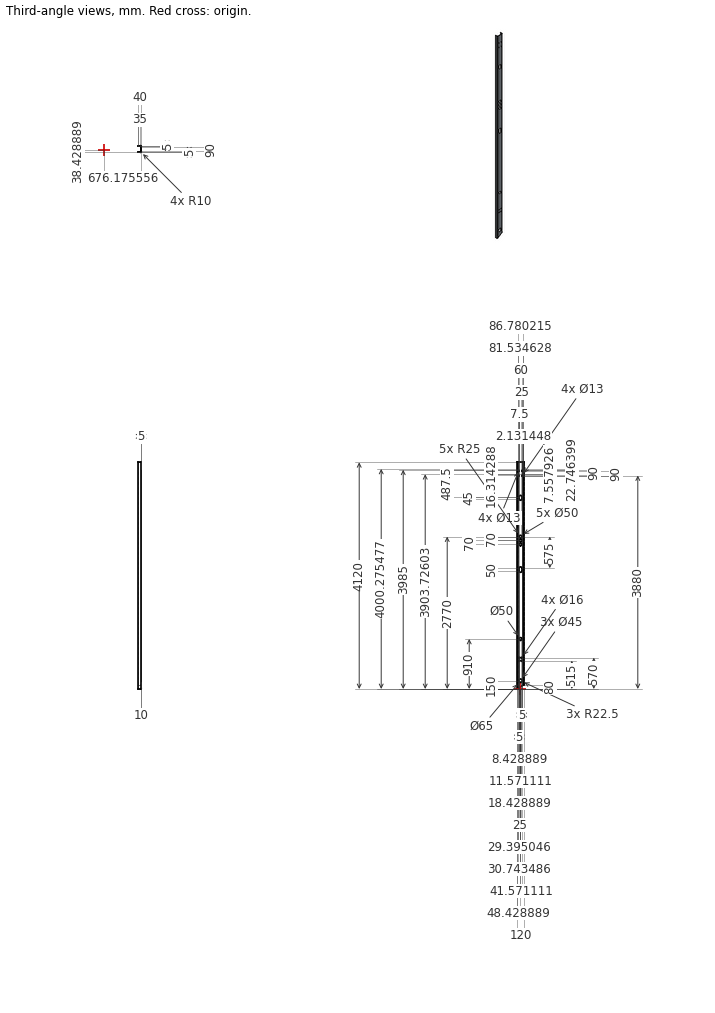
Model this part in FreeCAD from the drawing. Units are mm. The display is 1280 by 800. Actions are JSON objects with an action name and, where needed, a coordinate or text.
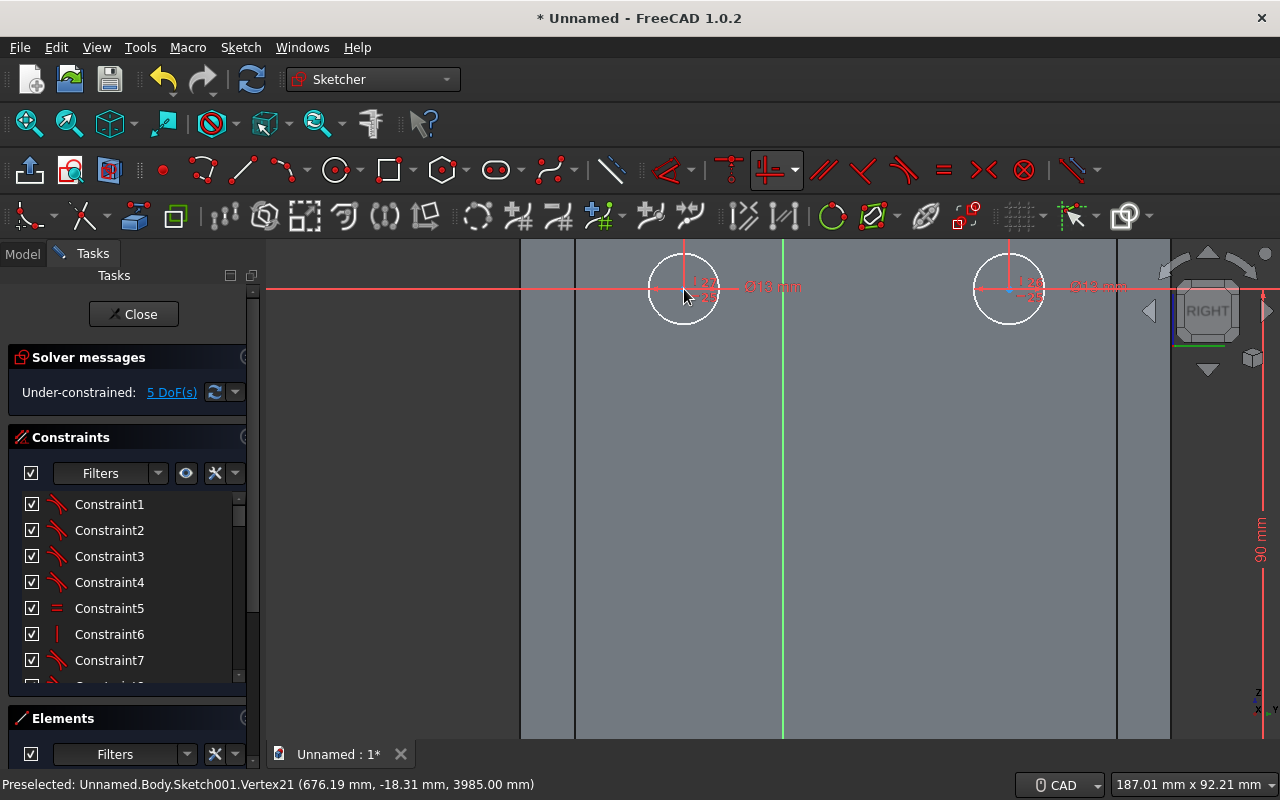
{"action": "scroll", "coordinate": [704, 489], "scroll_direction": "down", "scroll_amount": 15}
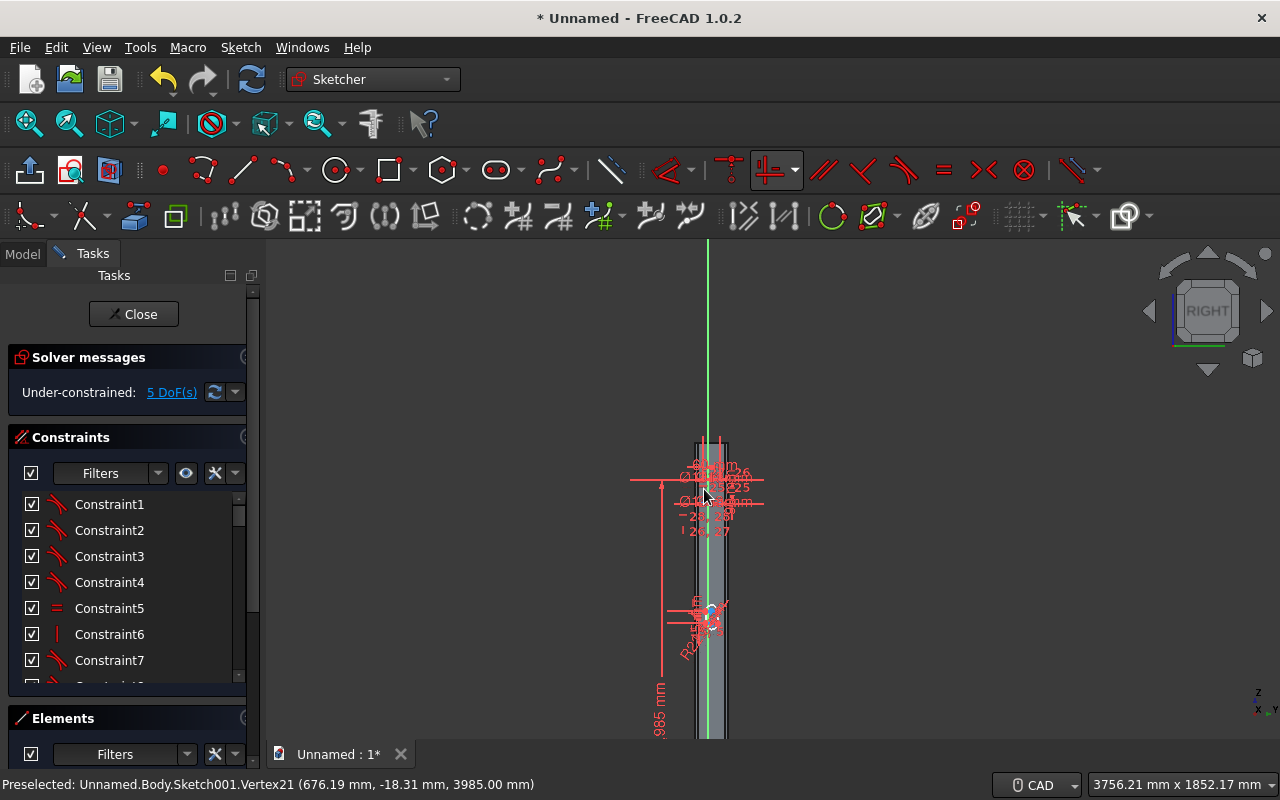
{"action": "scroll", "coordinate": [701, 267], "scroll_direction": "down", "scroll_amount": 6}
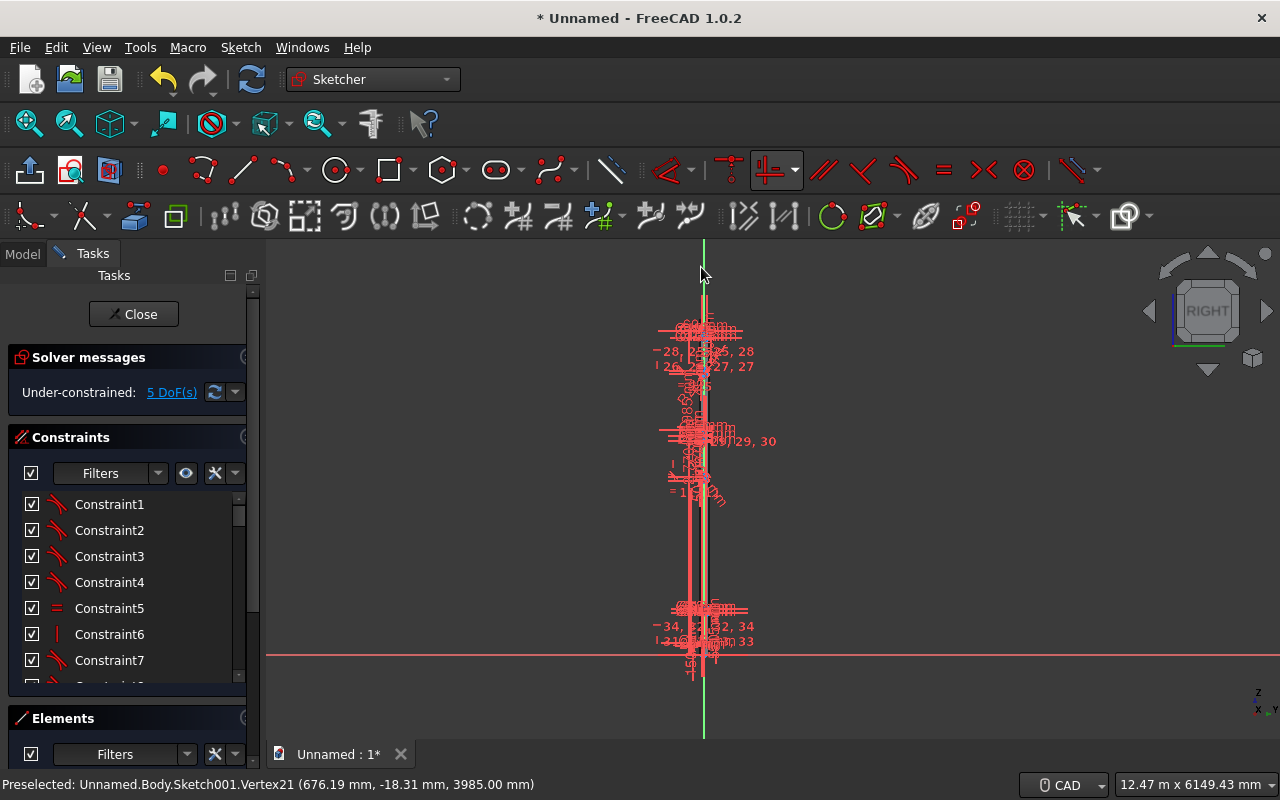
{"action": "scroll", "coordinate": [703, 371], "scroll_direction": "up", "scroll_amount": 21}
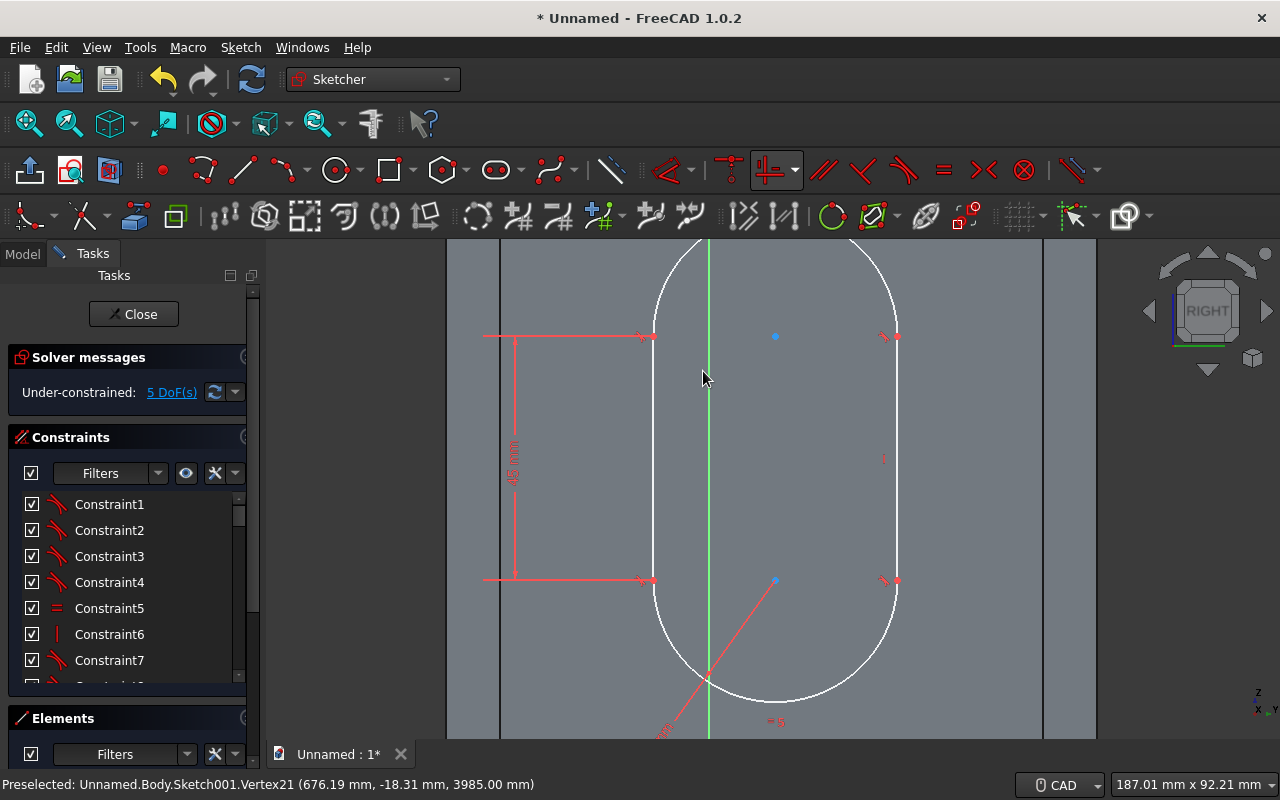
{"action": "left_click", "coordinate": [653, 336]}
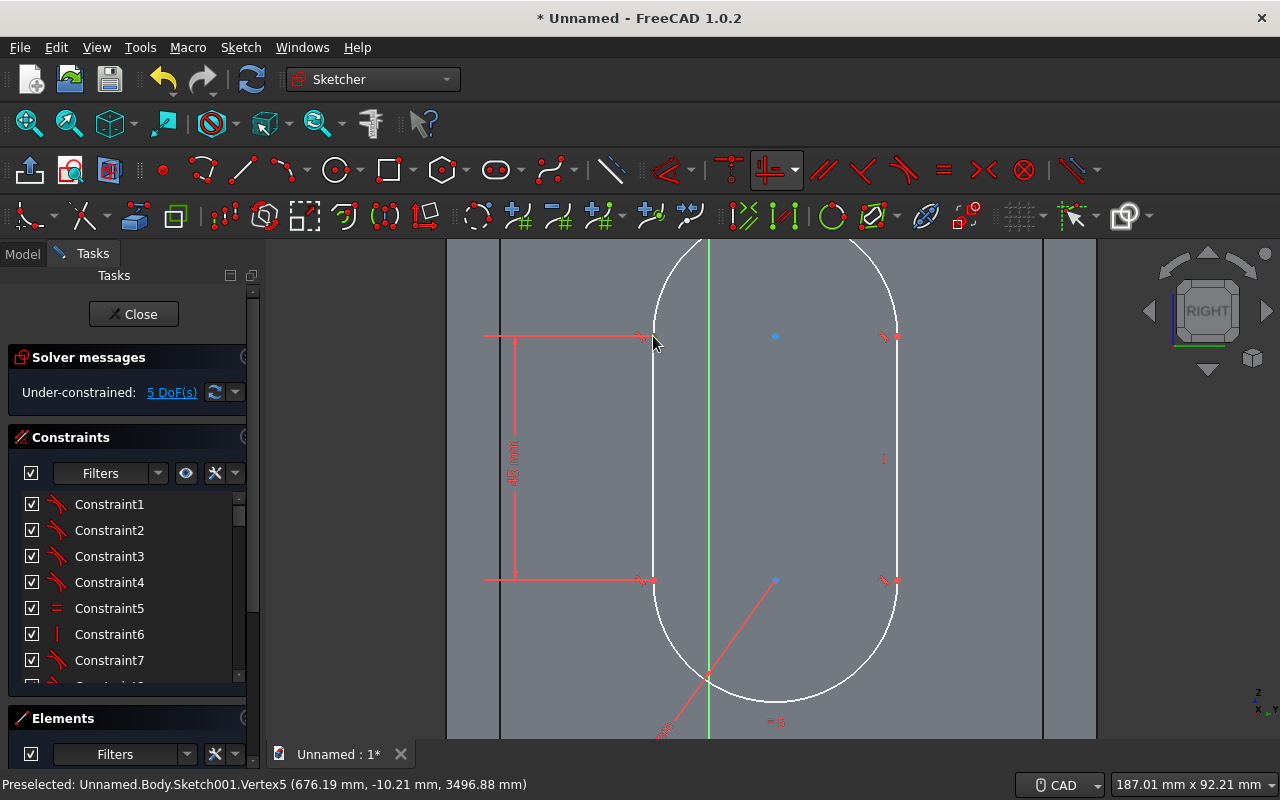
{"action": "scroll", "coordinate": [704, 489], "scroll_direction": "down", "scroll_amount": 15}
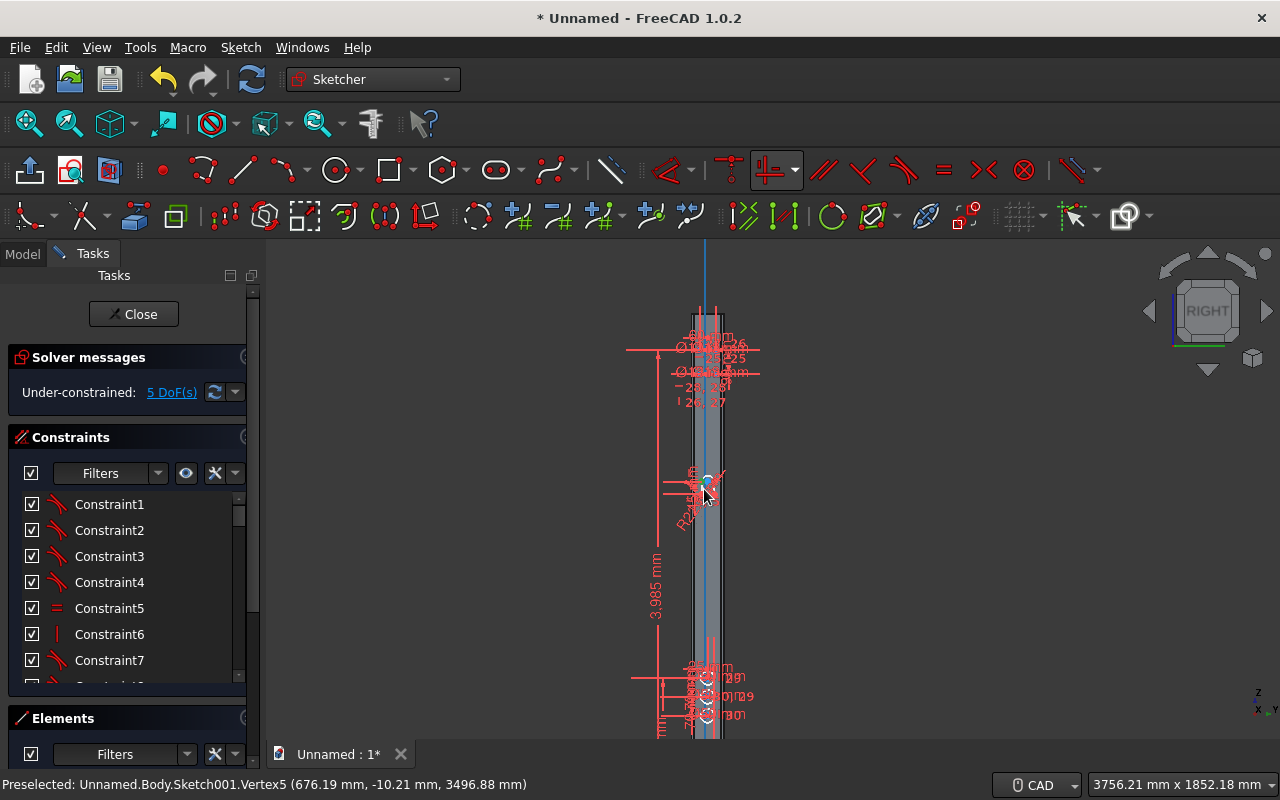
{"action": "scroll", "coordinate": [703, 317], "scroll_direction": "down", "scroll_amount": 6}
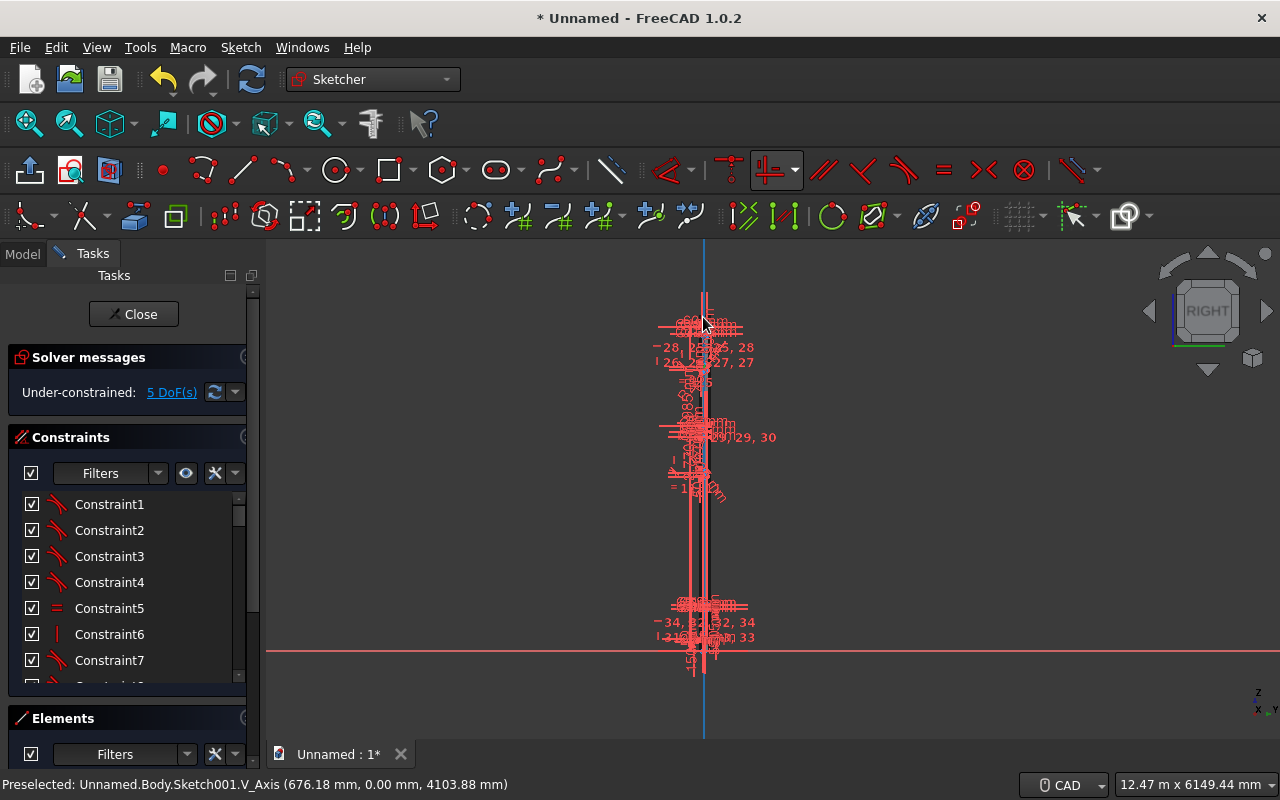
{"action": "scroll", "coordinate": [702, 327], "scroll_direction": "up", "scroll_amount": 21}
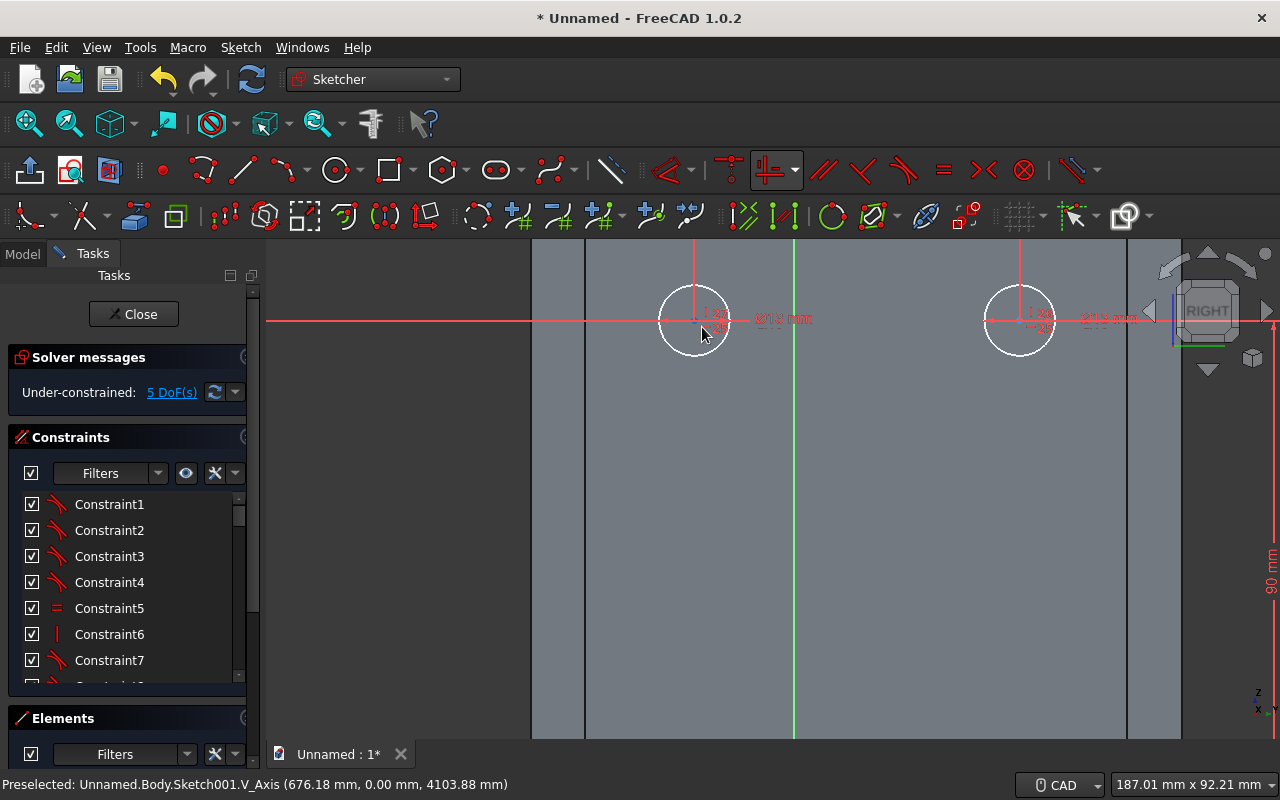
{"action": "left_click", "coordinate": [694, 321]}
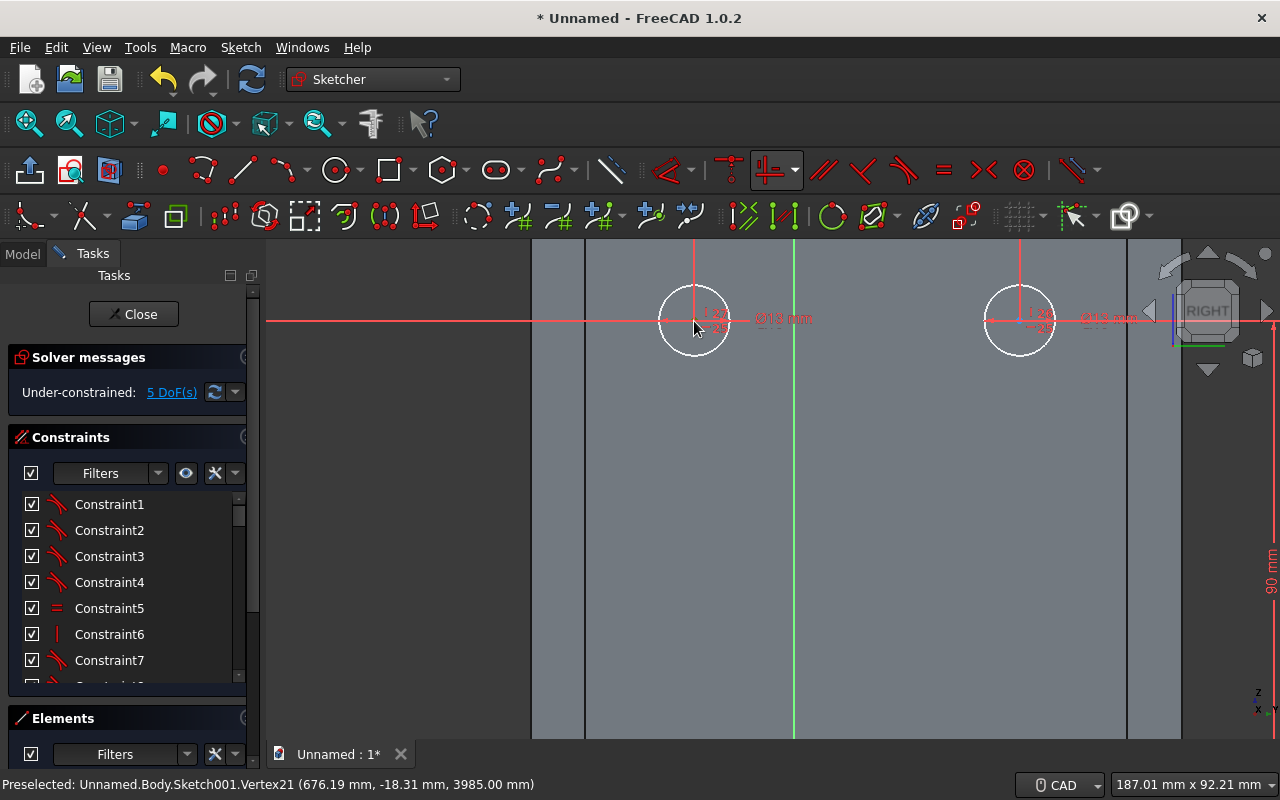
{"action": "key", "text": "l"}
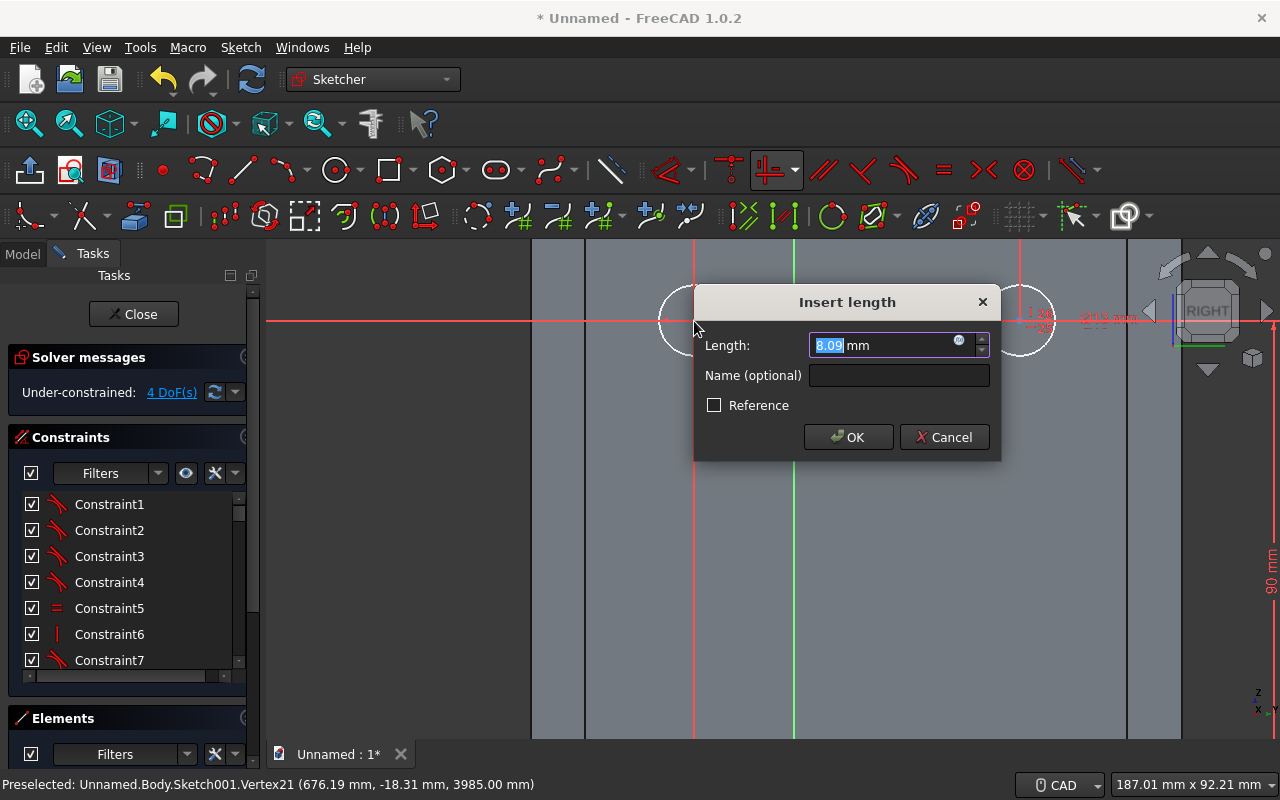
{"action": "type", "text": "7.5"}
{"action": "key", "text": "Return"}